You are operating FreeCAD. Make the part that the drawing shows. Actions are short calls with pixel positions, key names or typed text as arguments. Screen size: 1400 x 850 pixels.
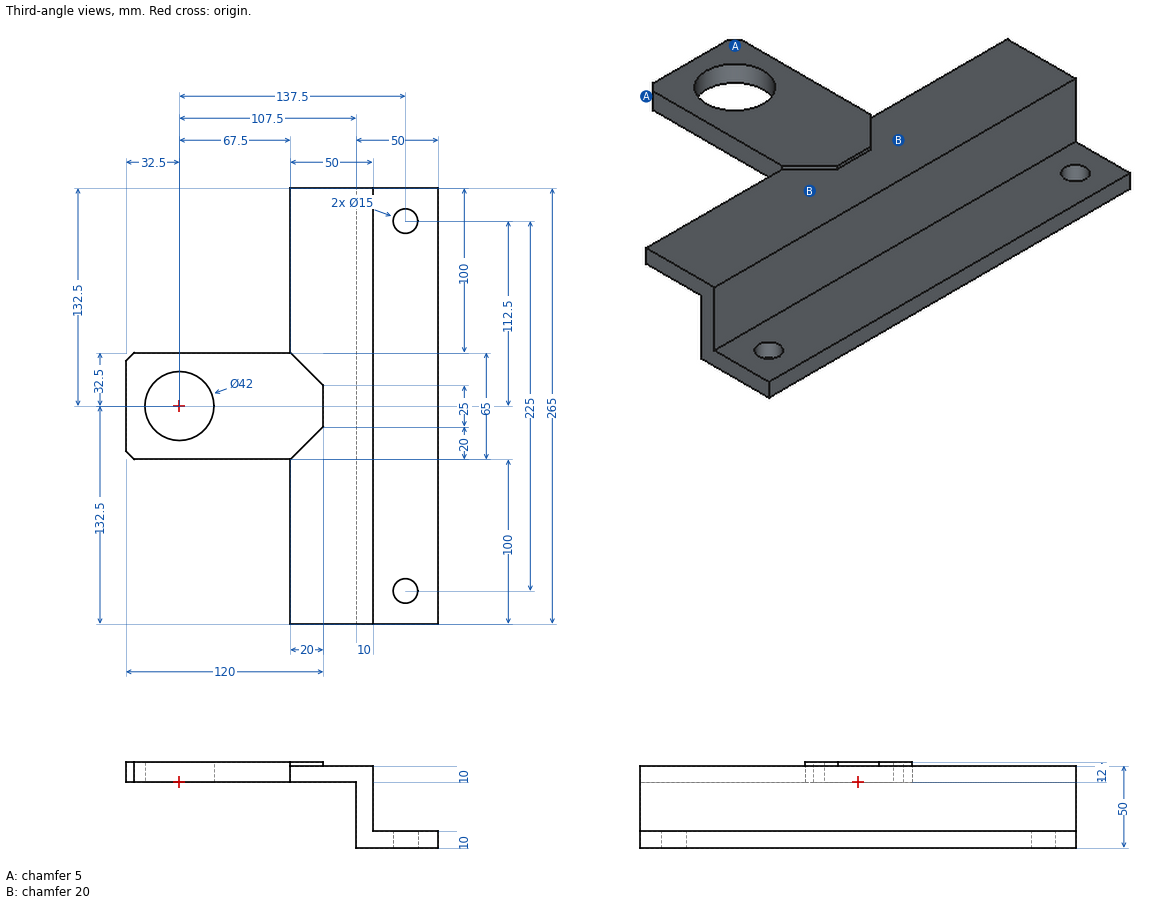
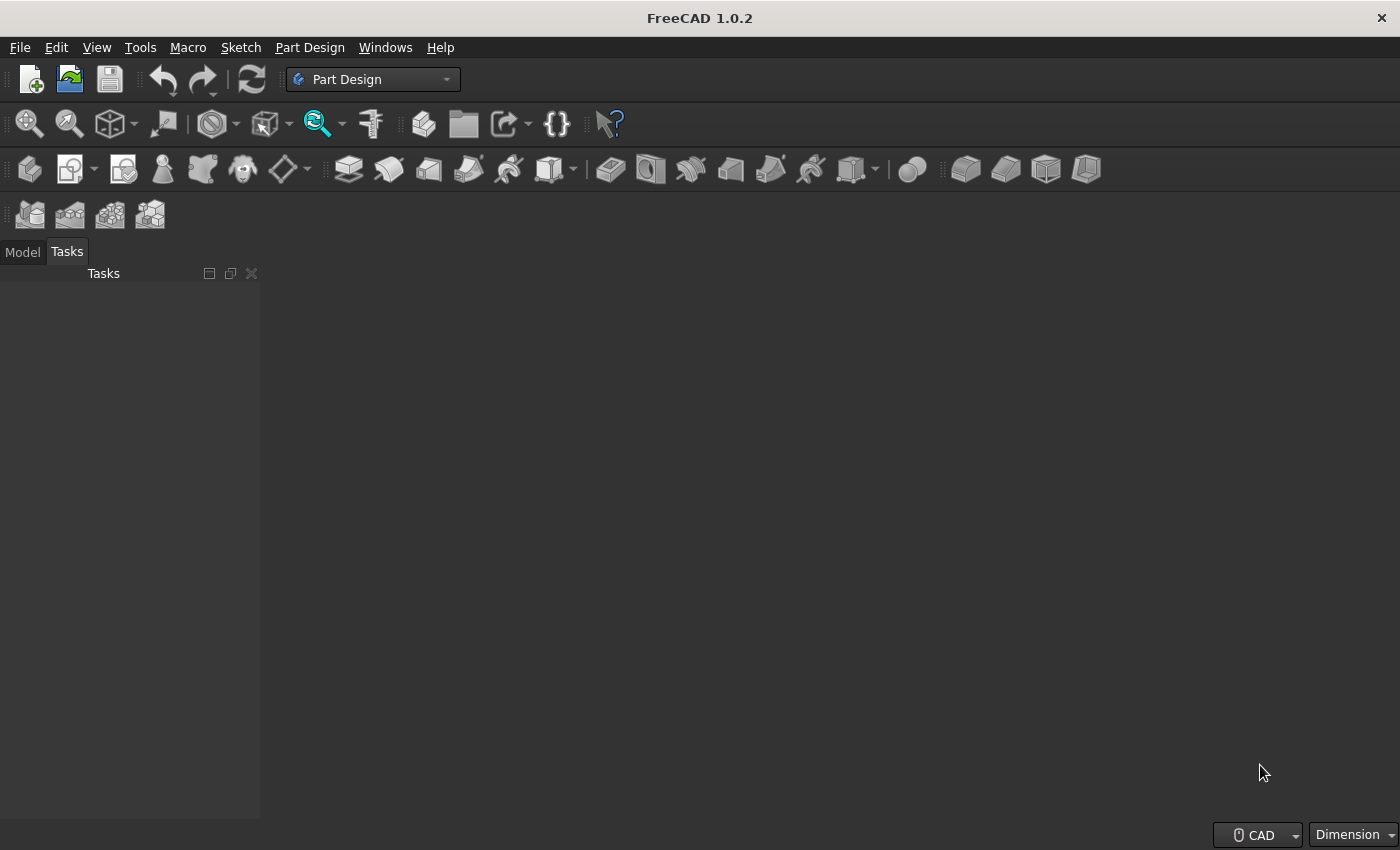
key(ctrl+n)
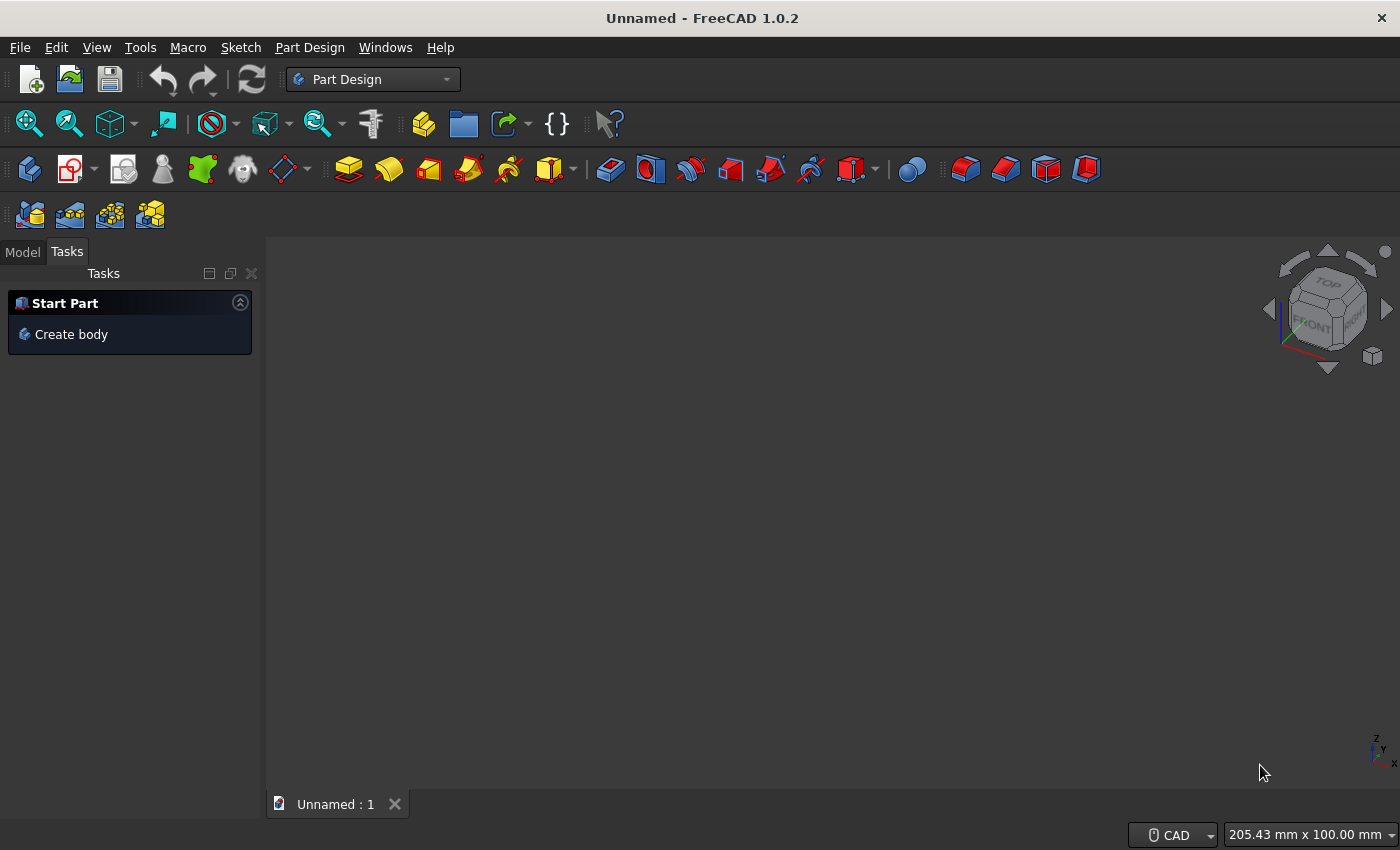
click(70, 170)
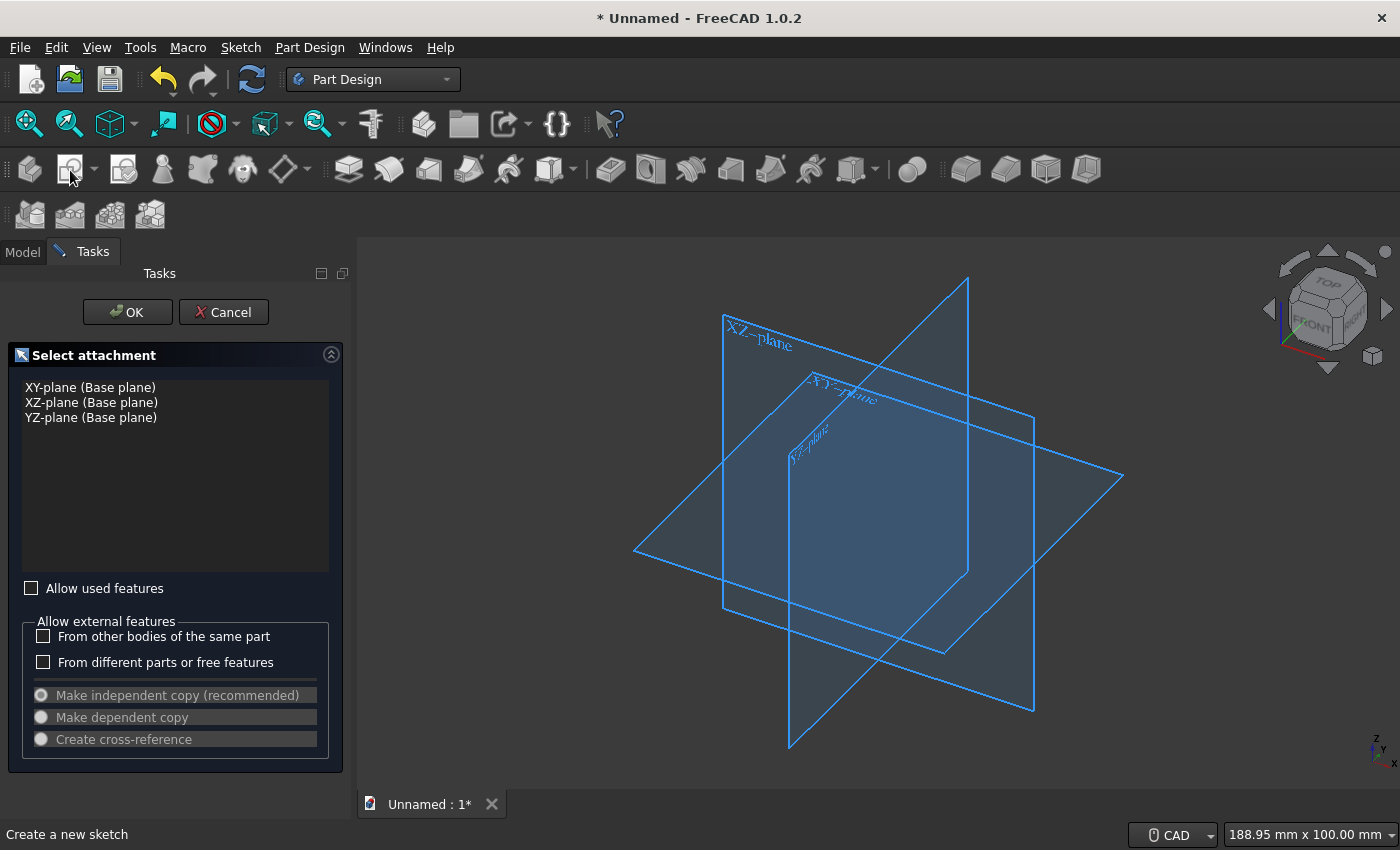
click(82, 388)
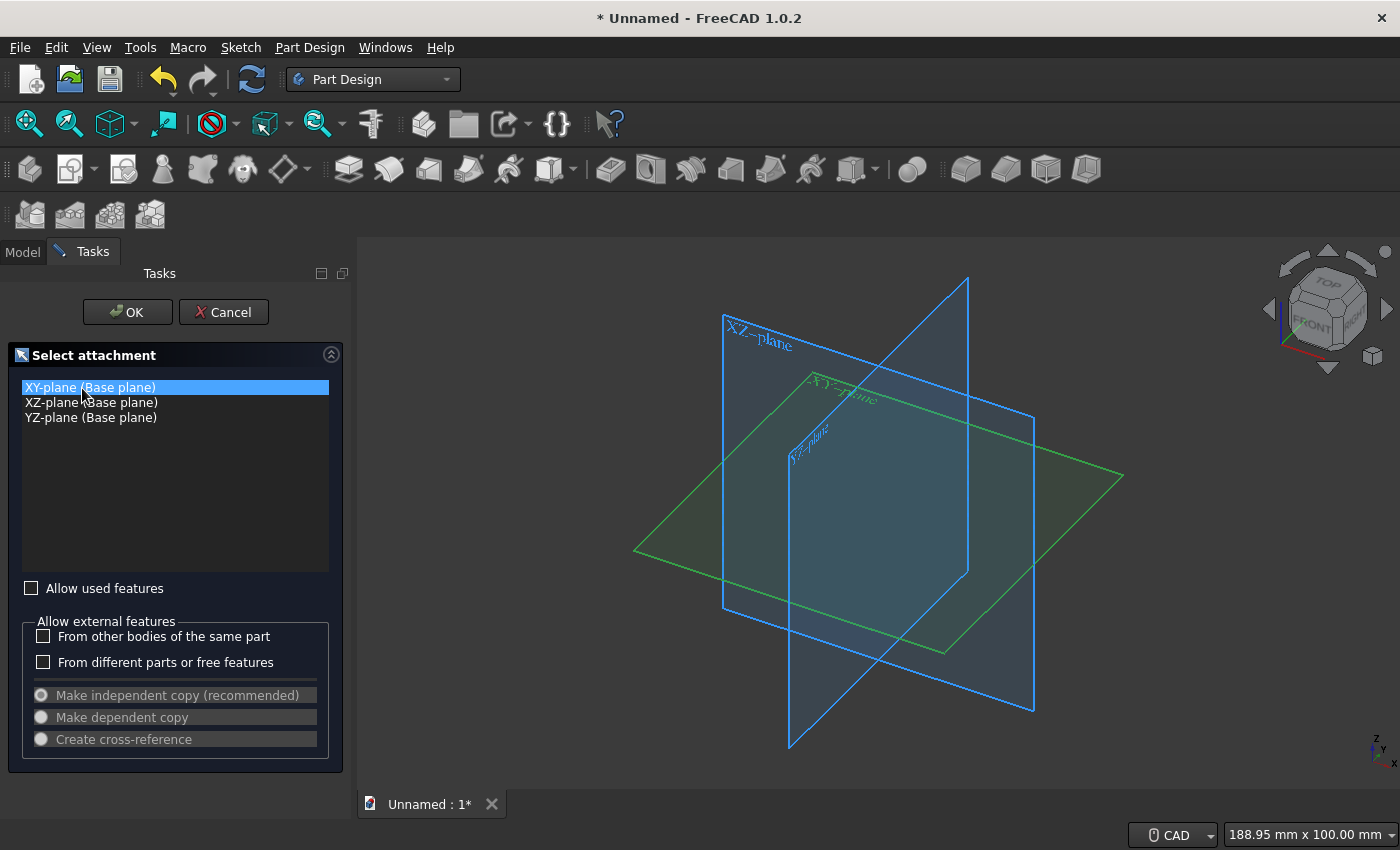
click(128, 312)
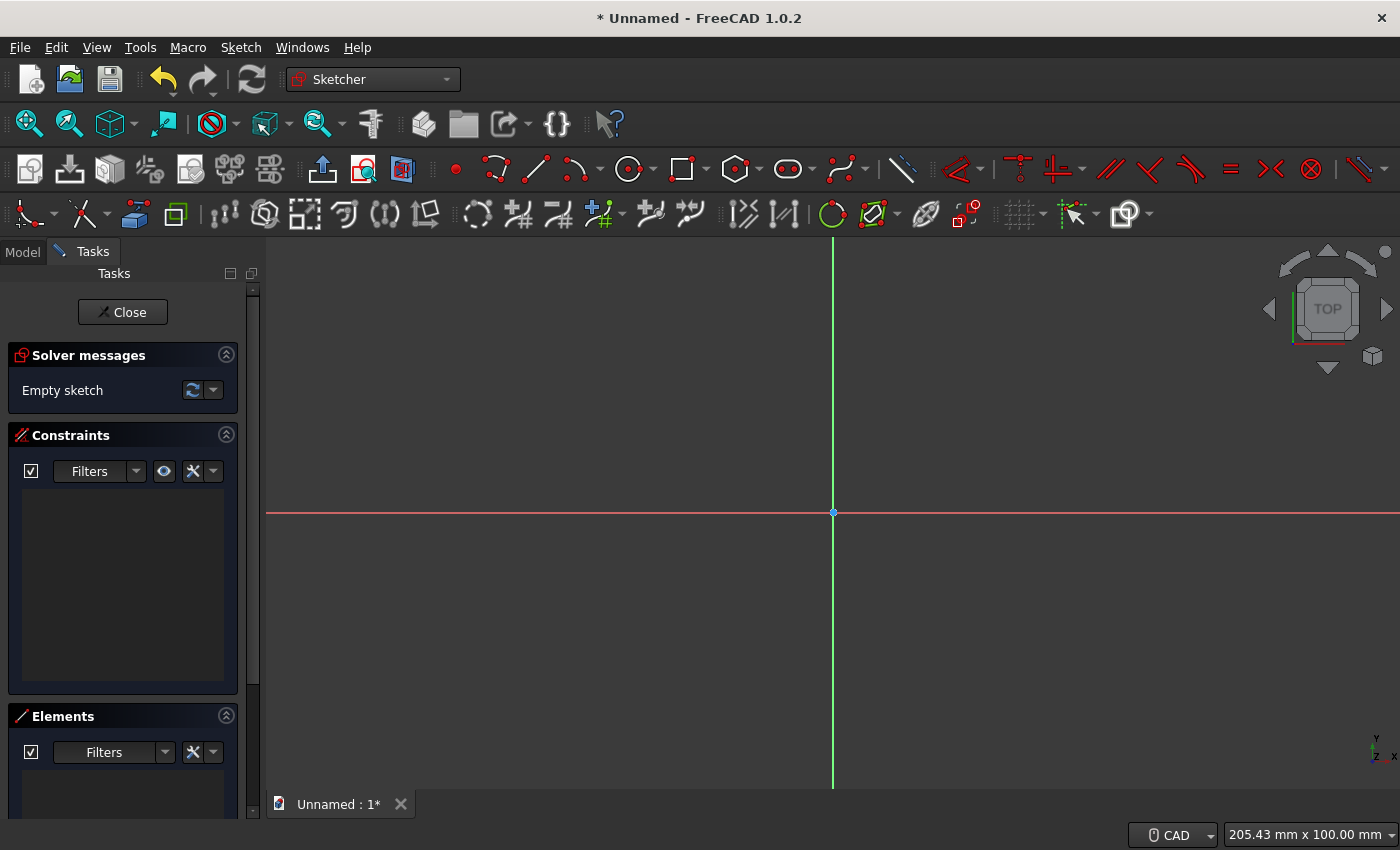
scroll(294, 513, down, 1)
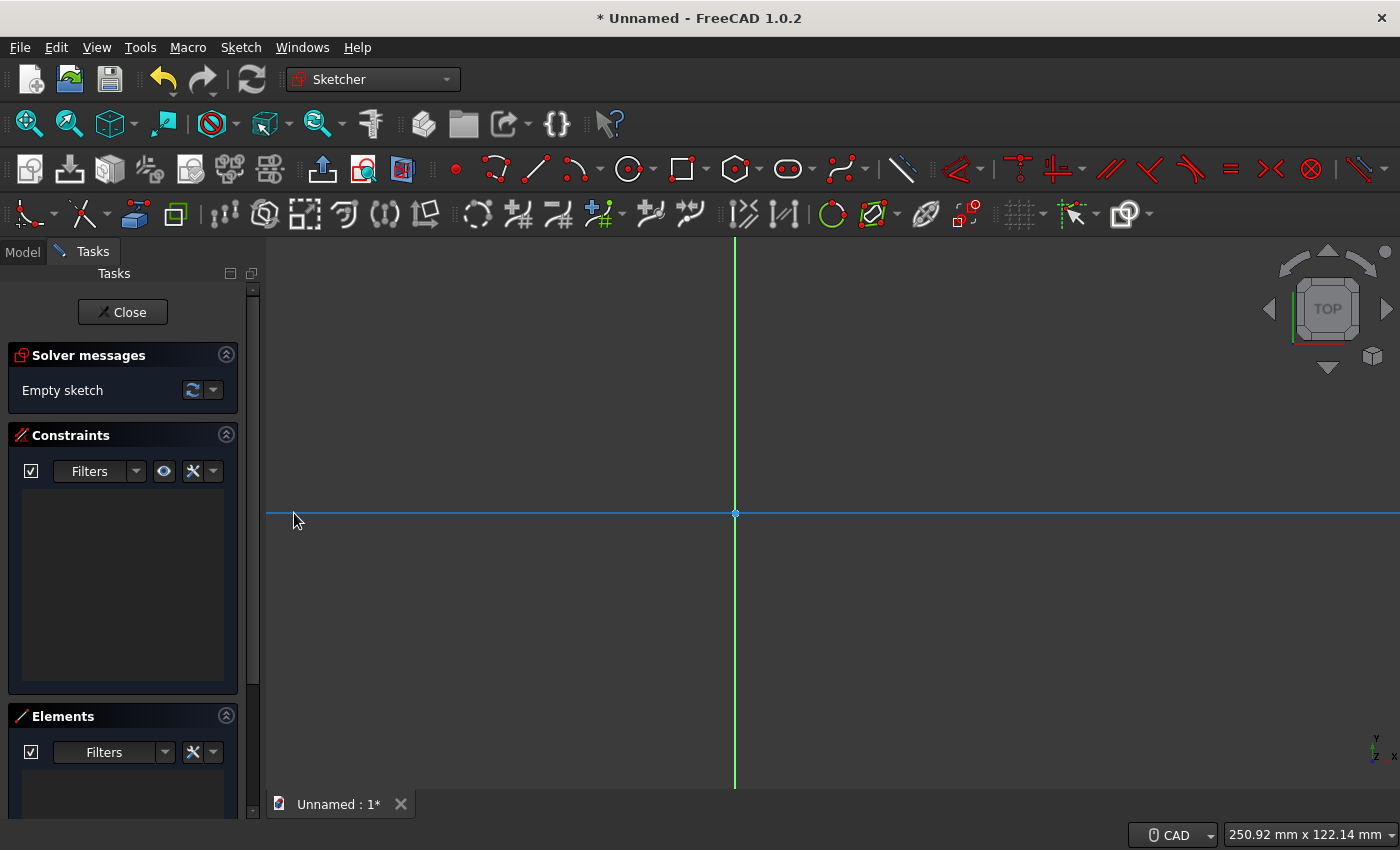
key(g)
key(r)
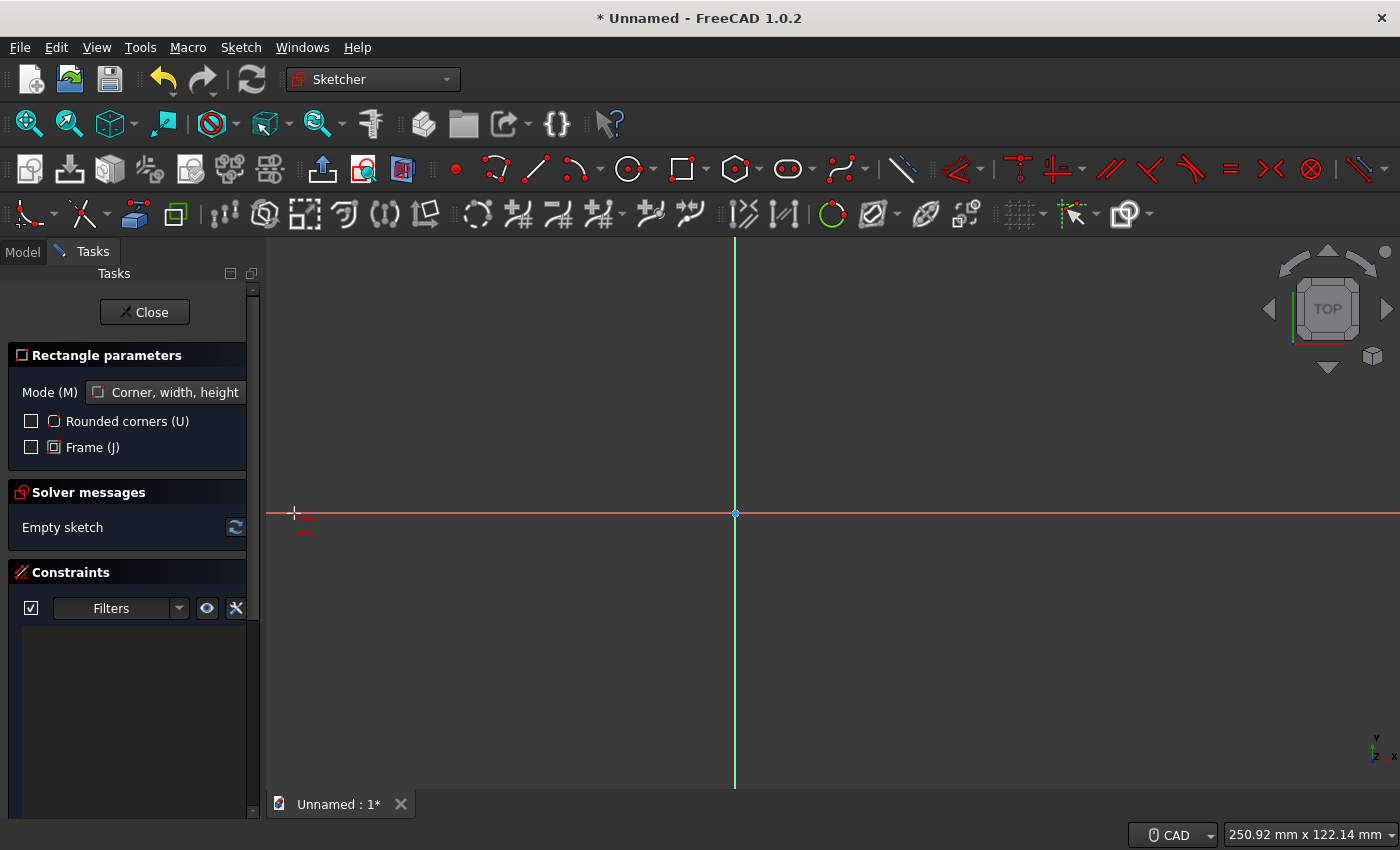
click(588, 366)
move(1131, 660)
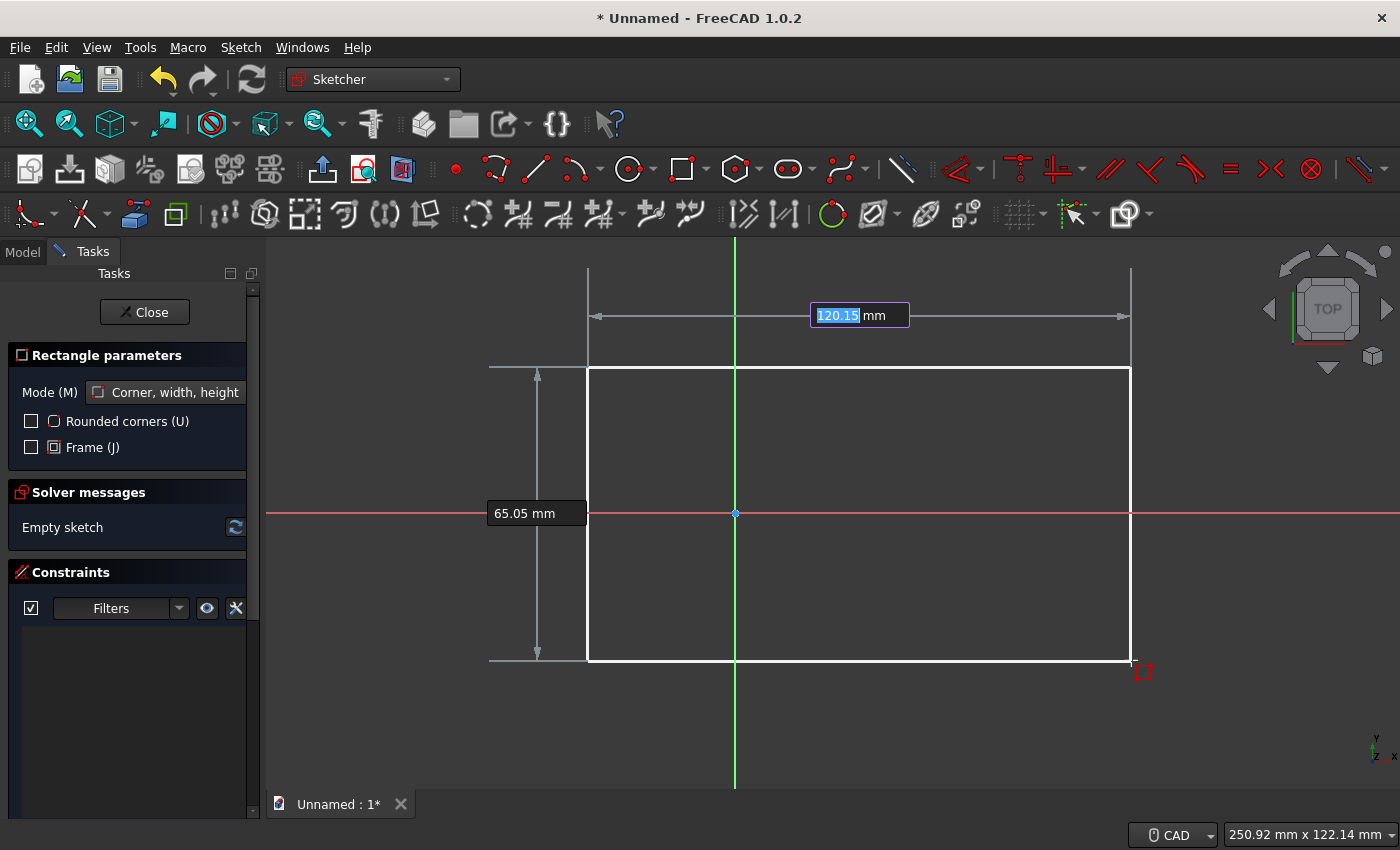
text(120)
key(Tab)
text(65)
key(Return)